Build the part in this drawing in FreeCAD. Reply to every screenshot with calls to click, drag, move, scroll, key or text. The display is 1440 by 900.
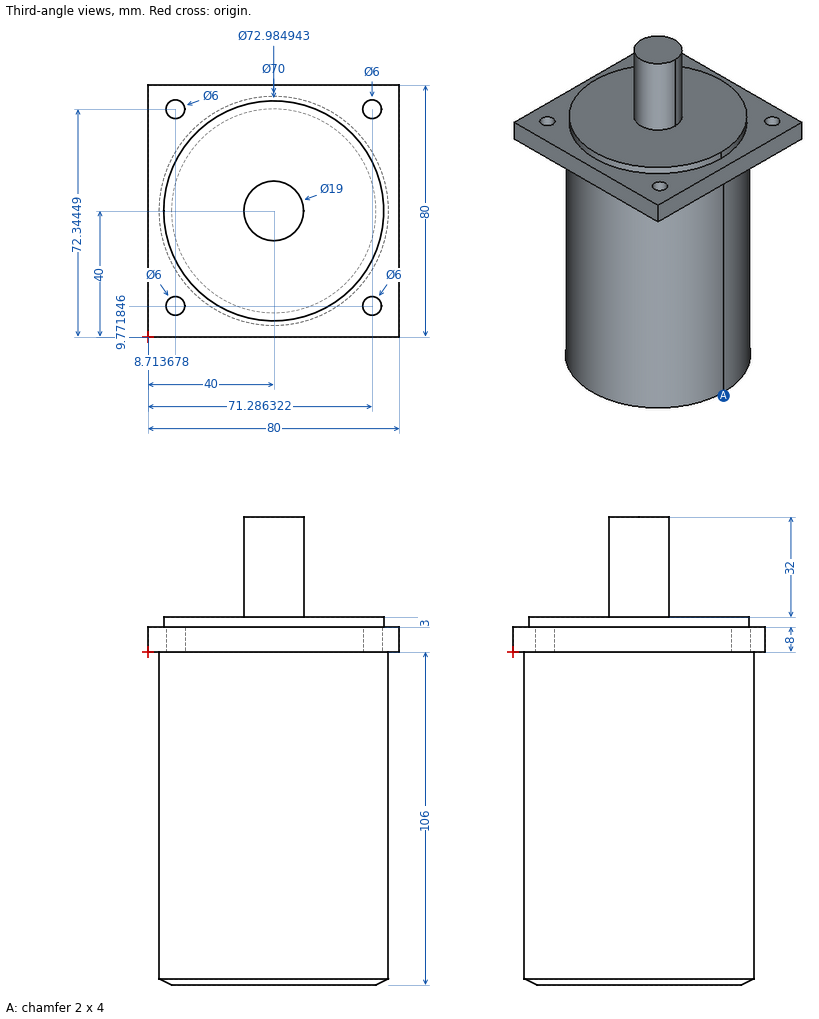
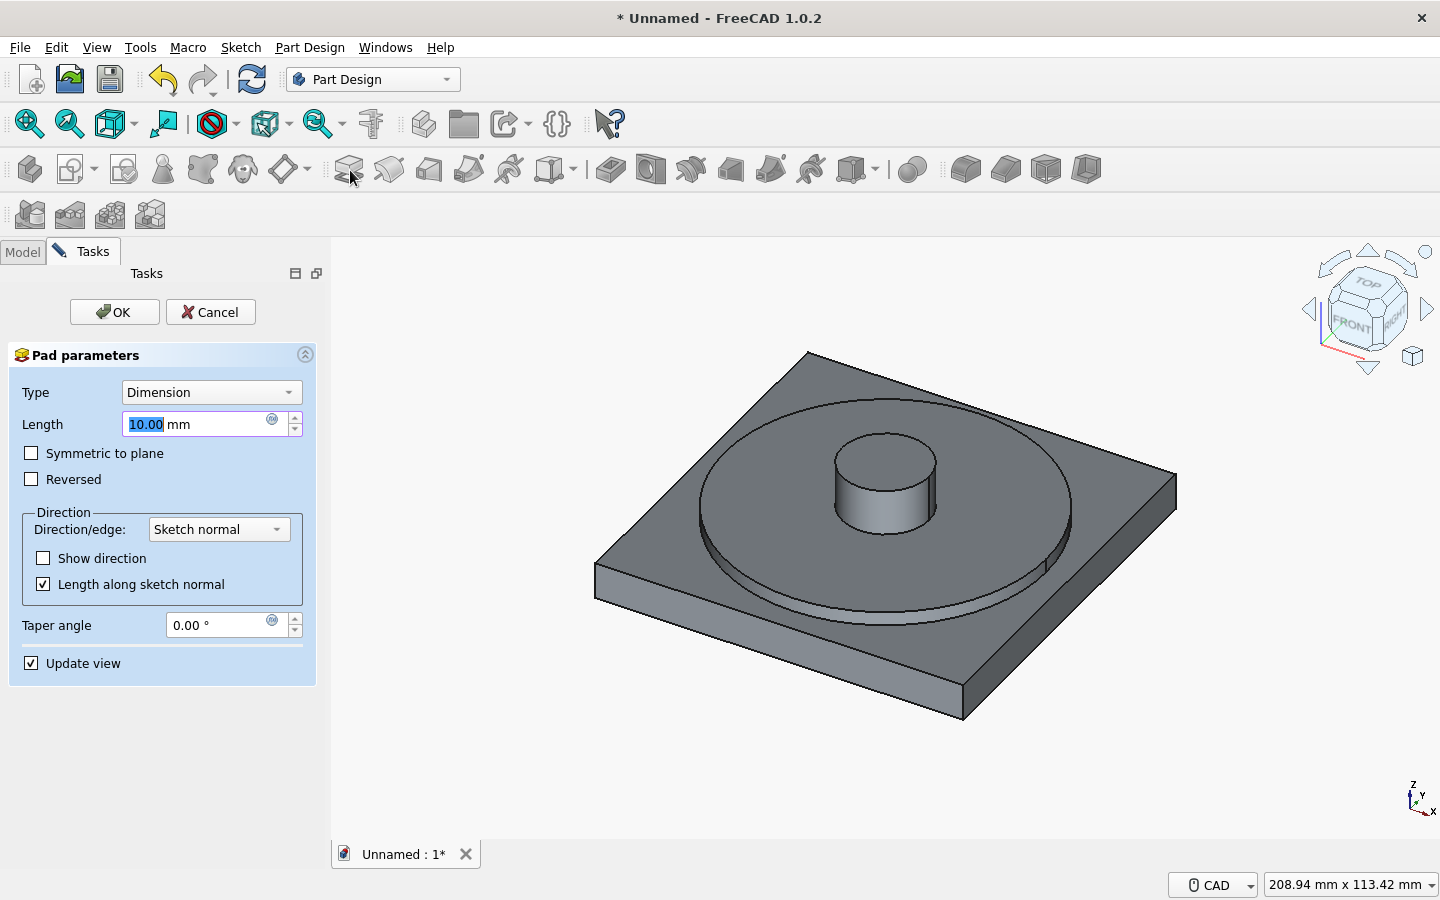
text(32)
key(Tab)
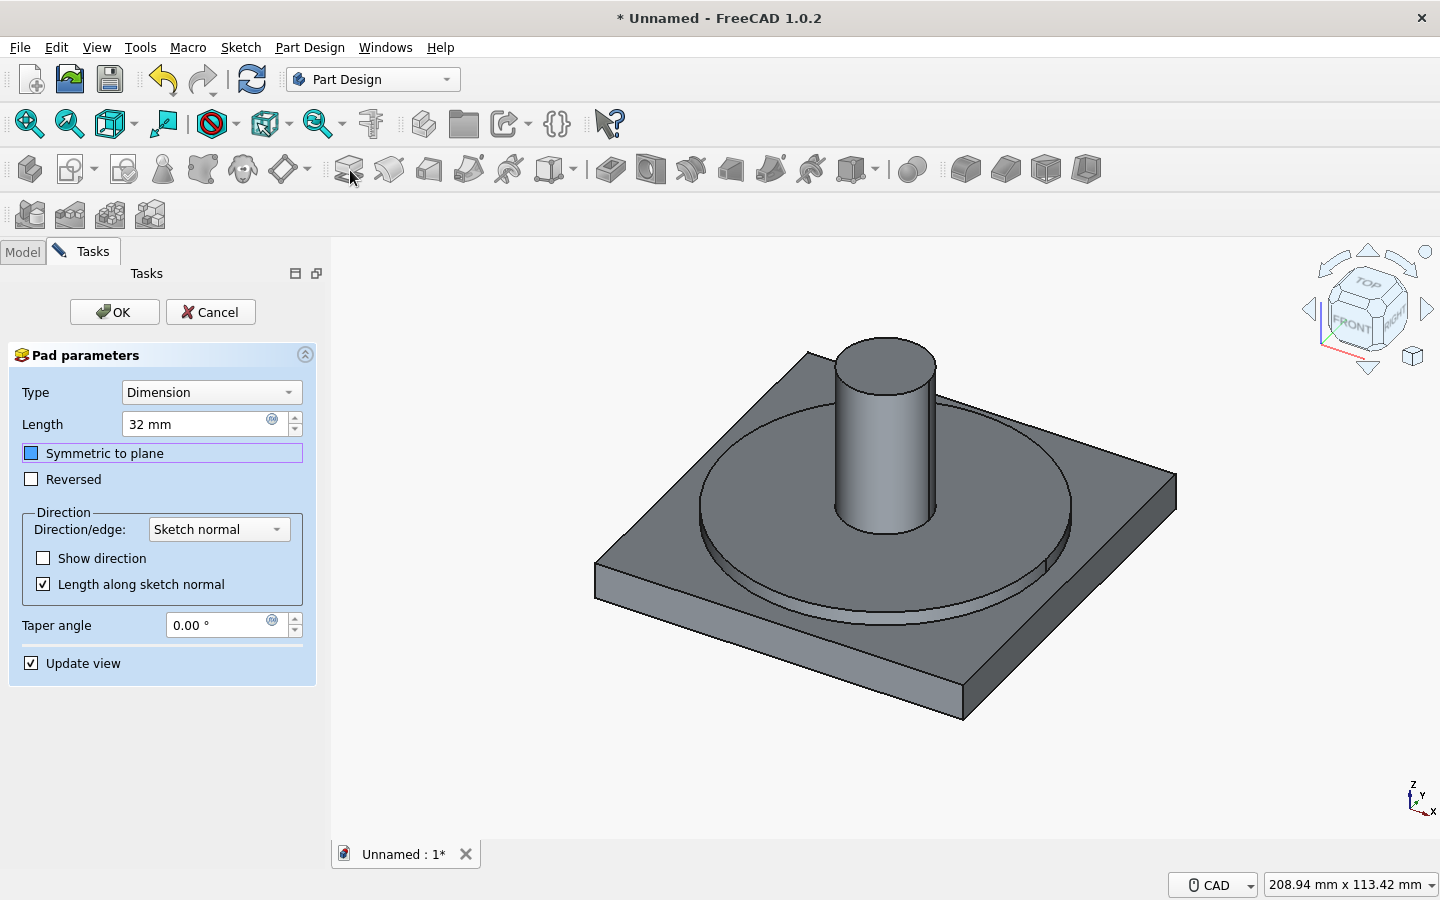
click(115, 312)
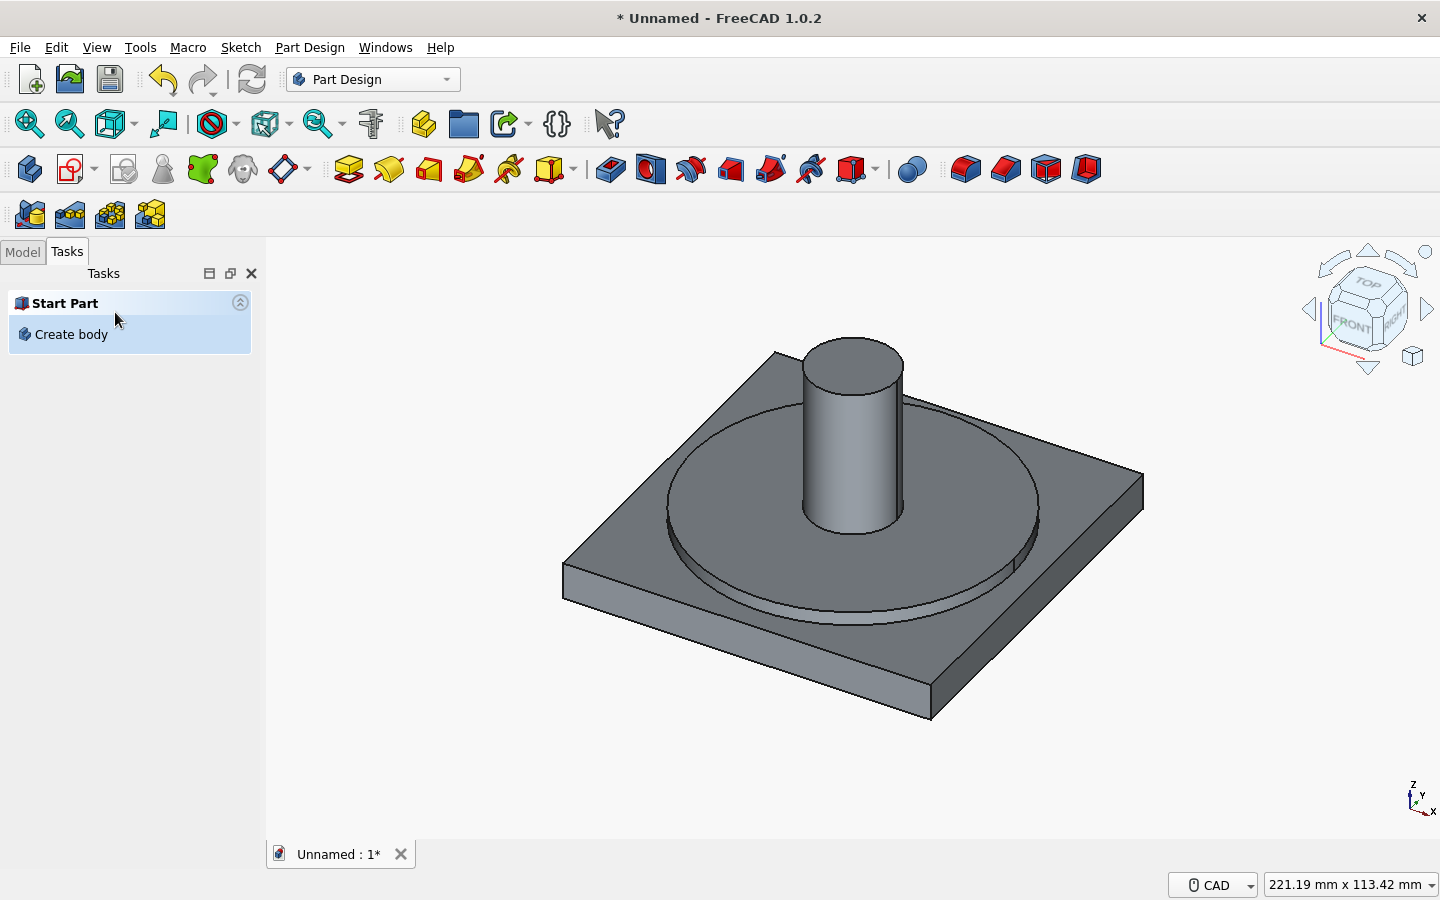
click(30, 124)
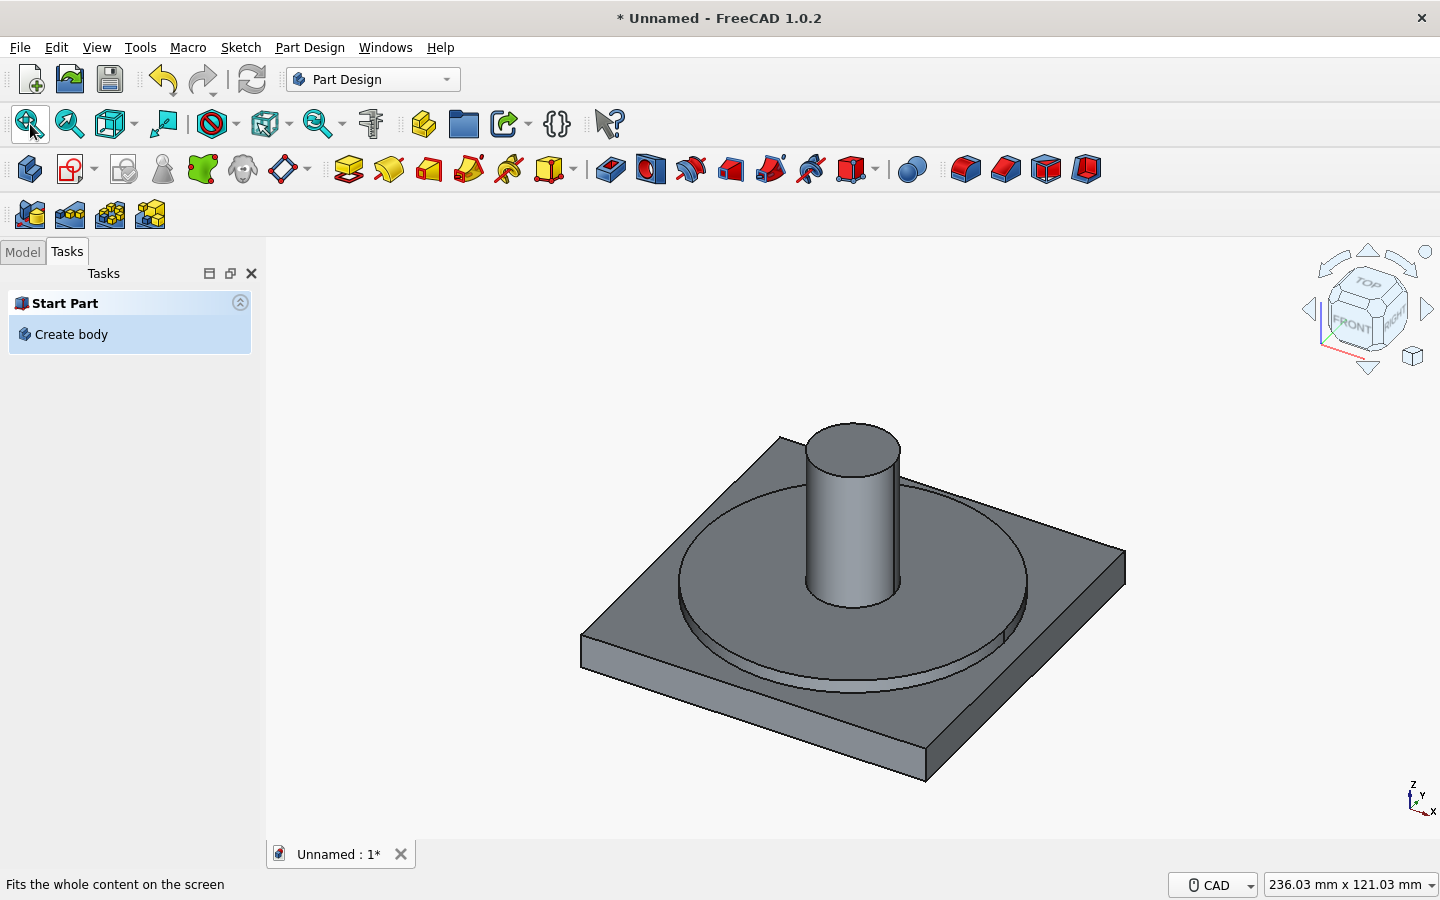
click(70, 170)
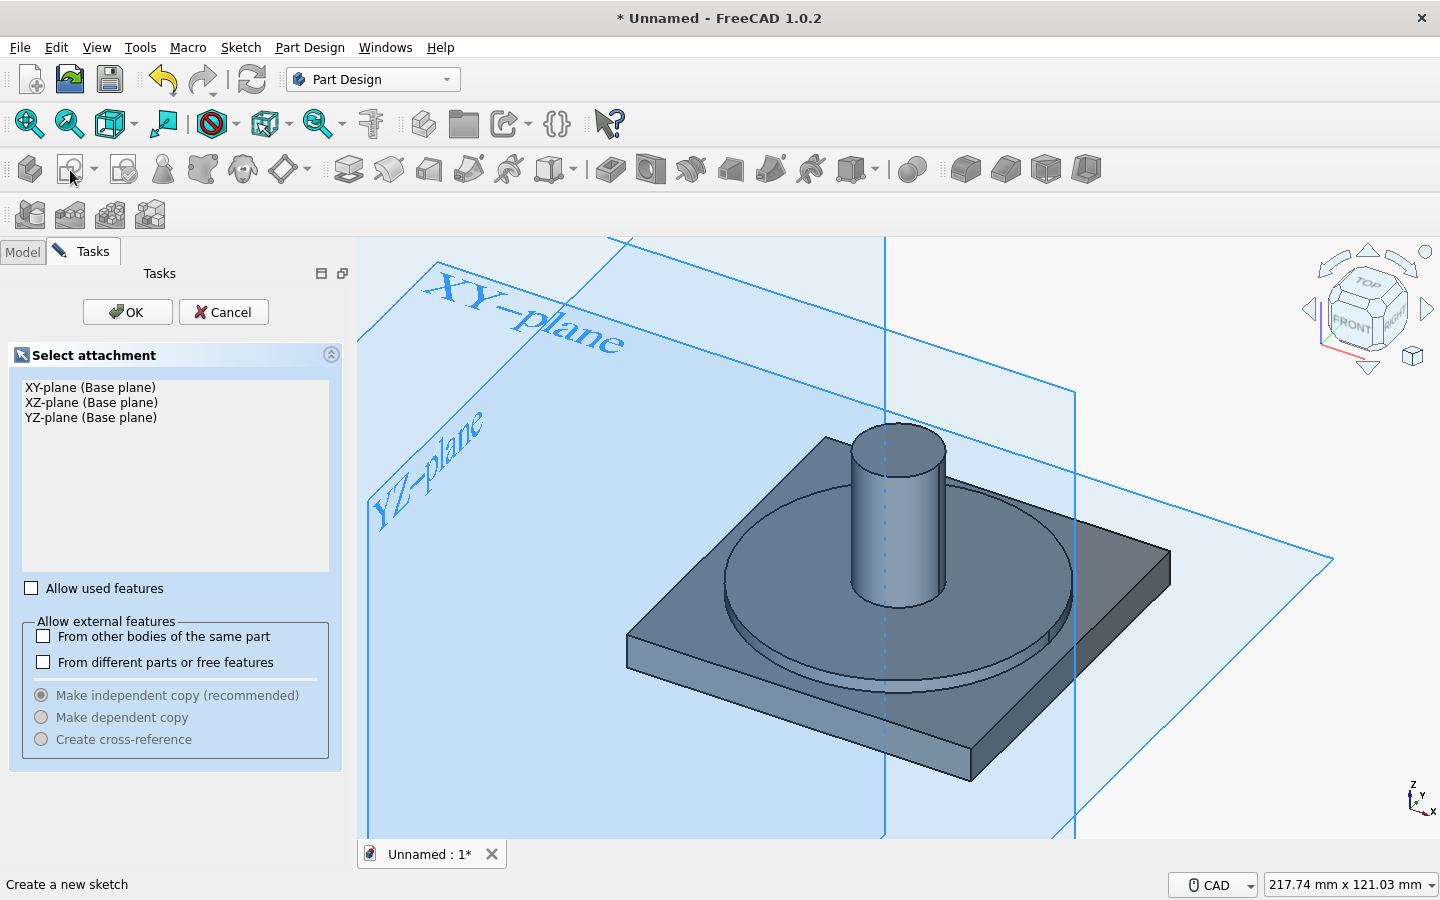
click(82, 388)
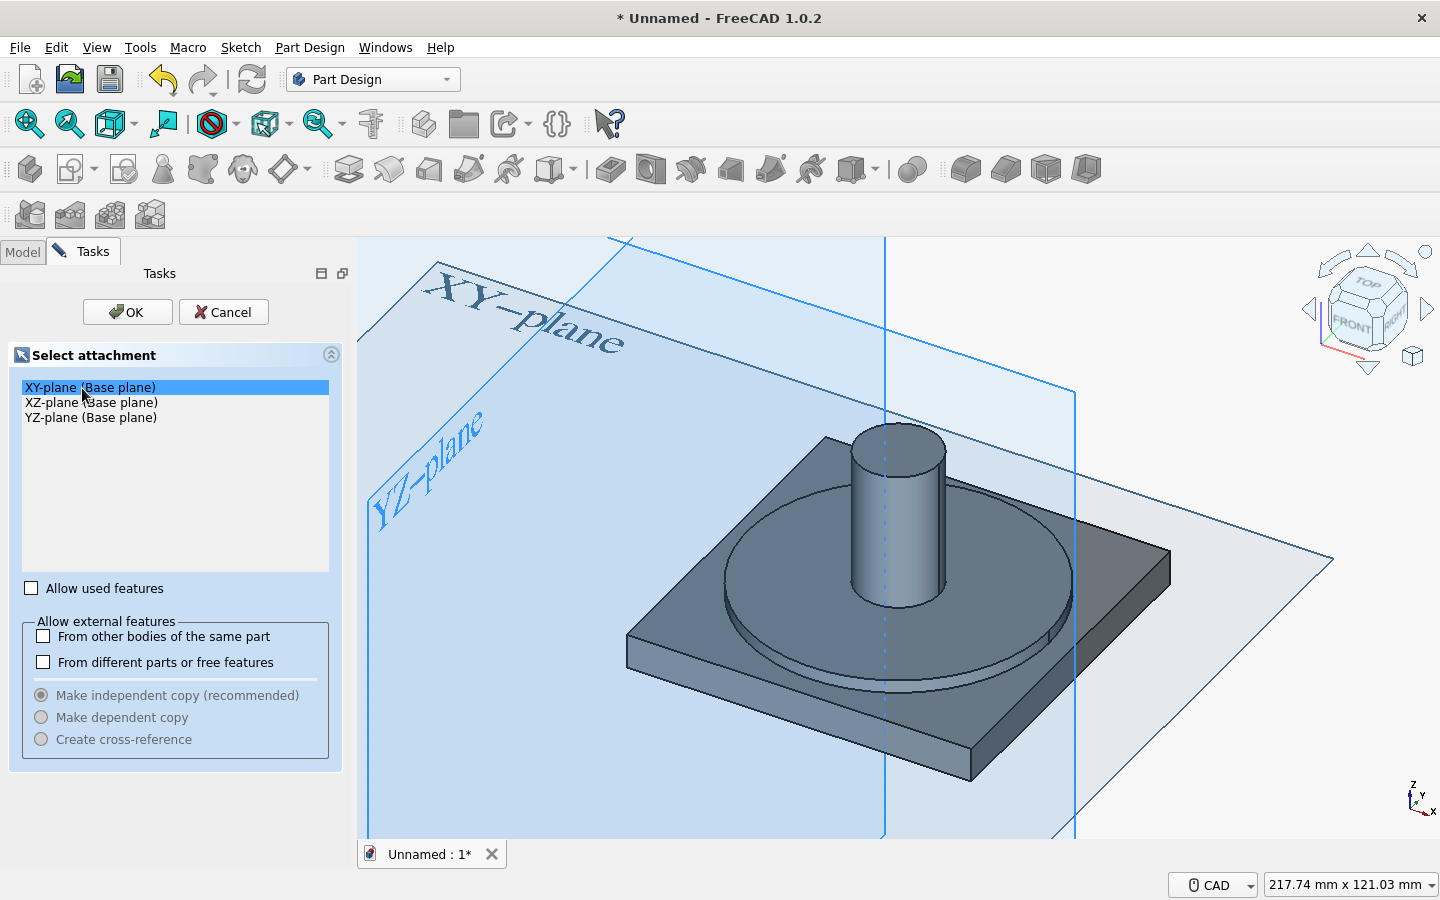
click(128, 312)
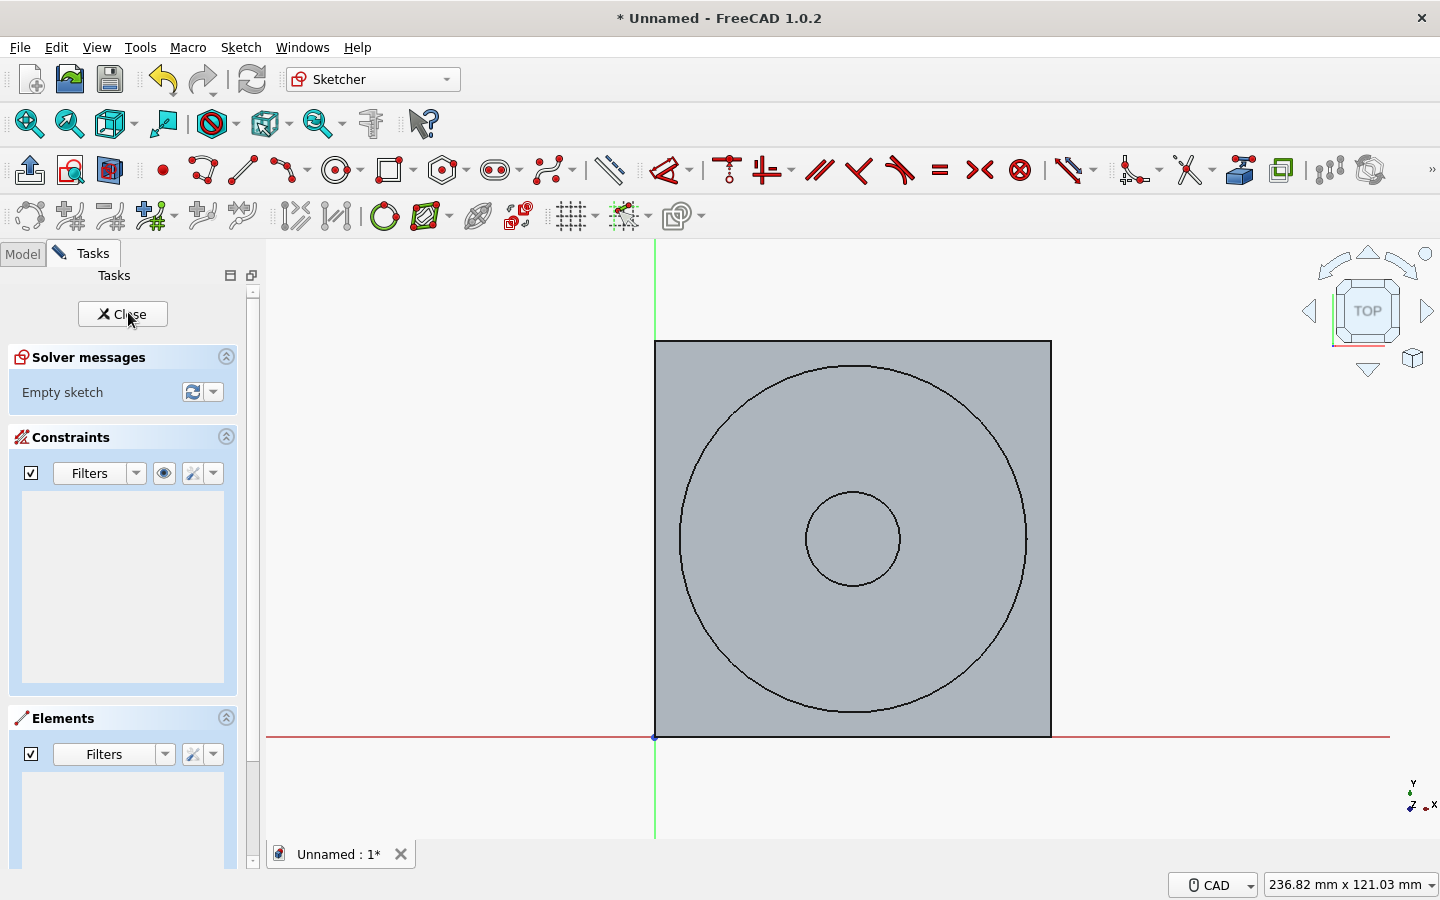
click(110, 170)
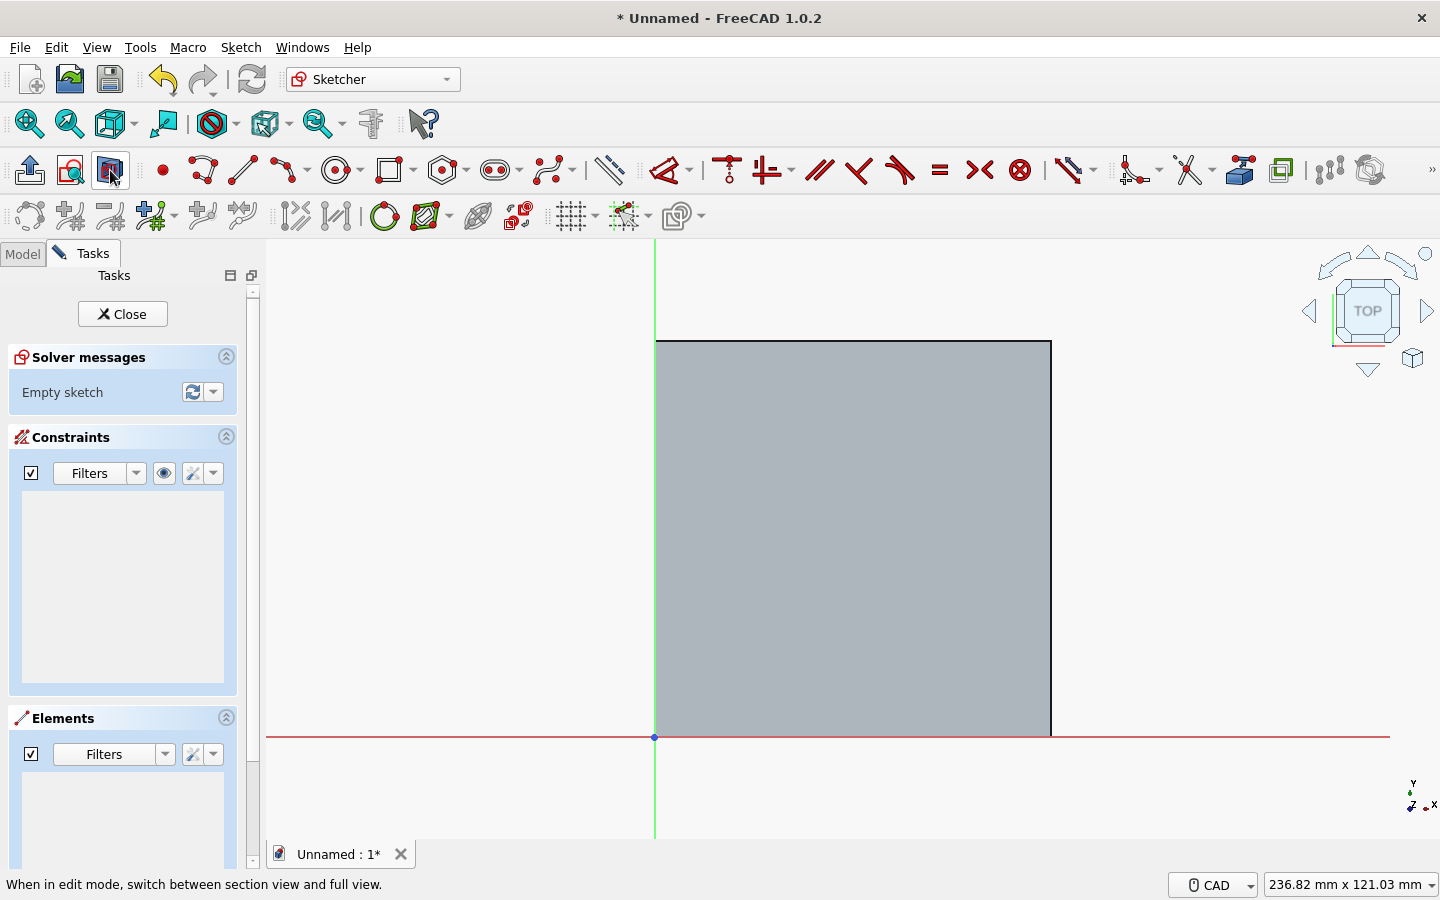
click(336, 170)